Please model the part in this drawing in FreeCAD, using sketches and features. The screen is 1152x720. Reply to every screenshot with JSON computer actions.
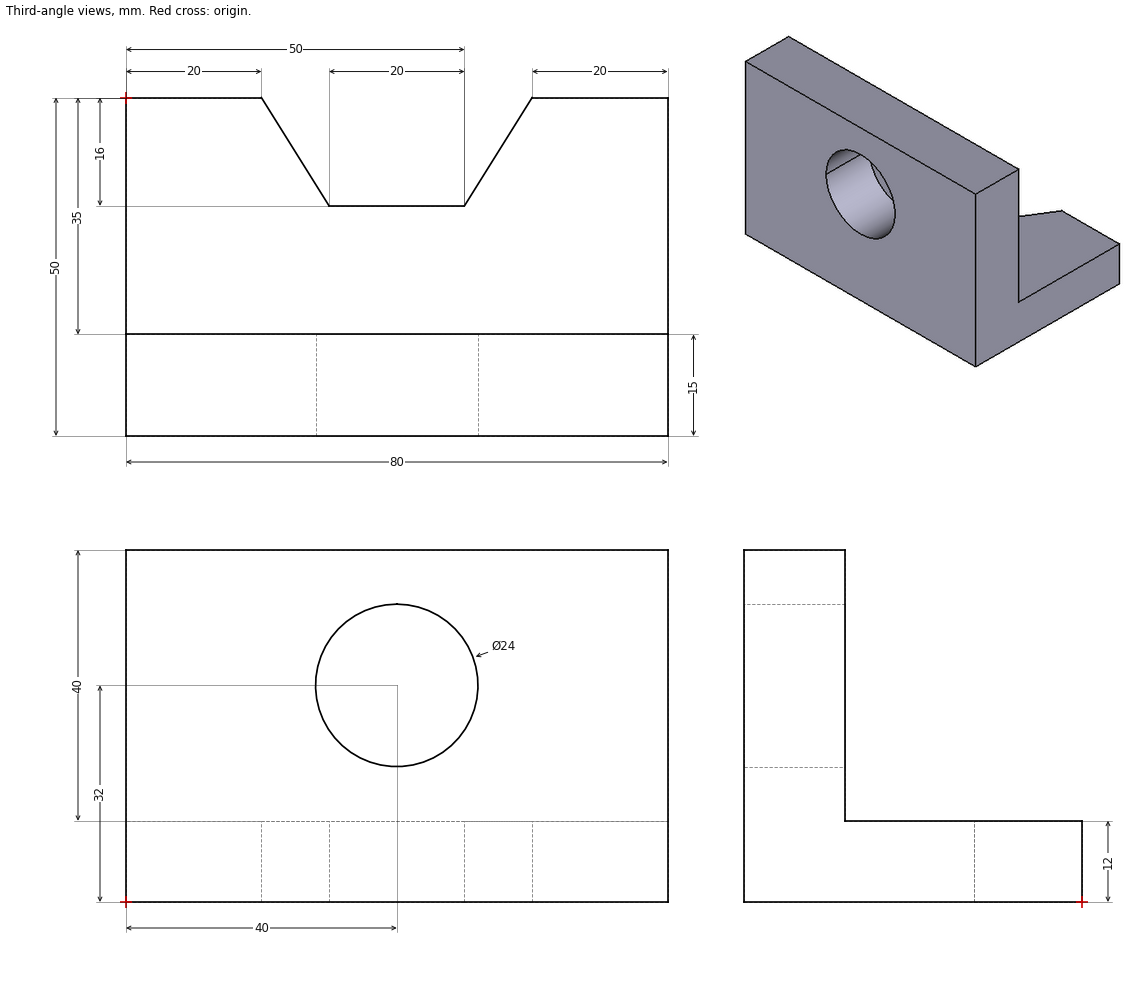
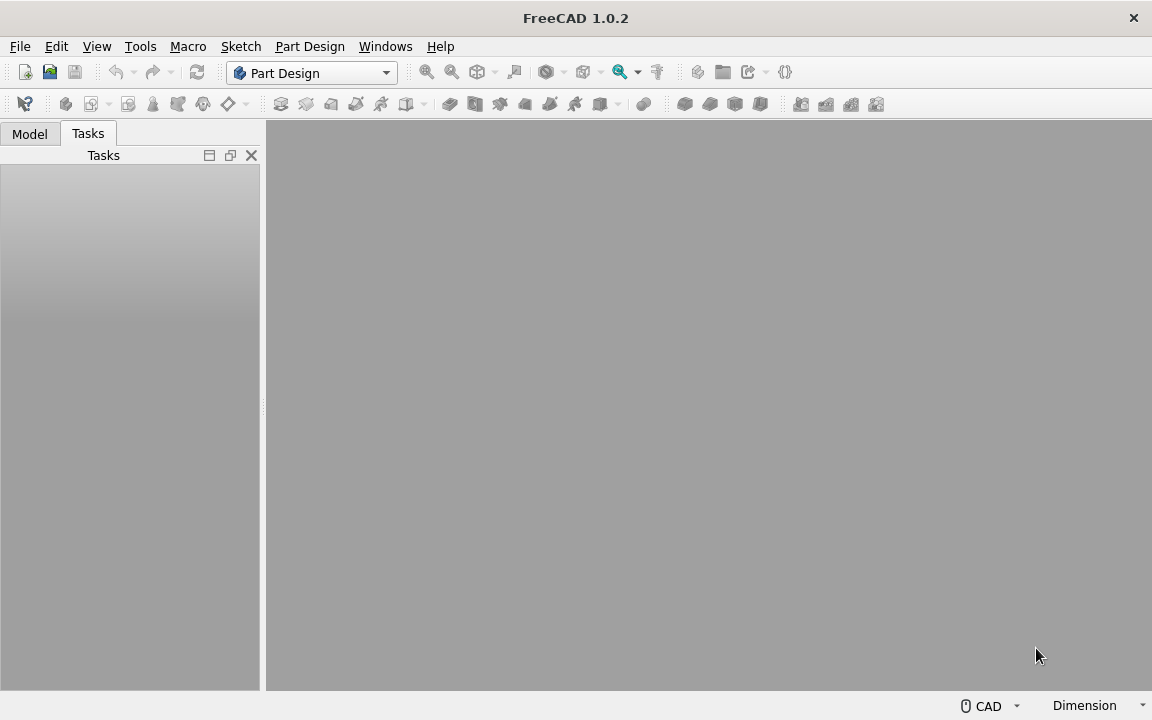
{"action": "key", "text": "ctrl+n"}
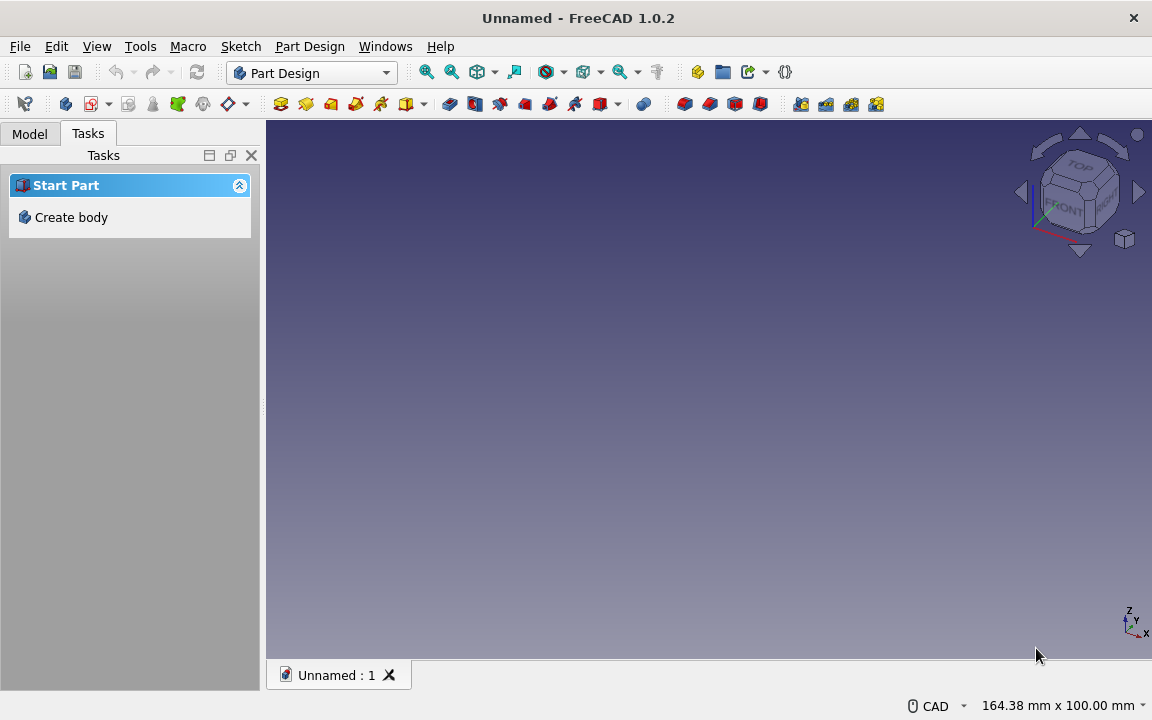
{"action": "left_click", "coordinate": [90, 104]}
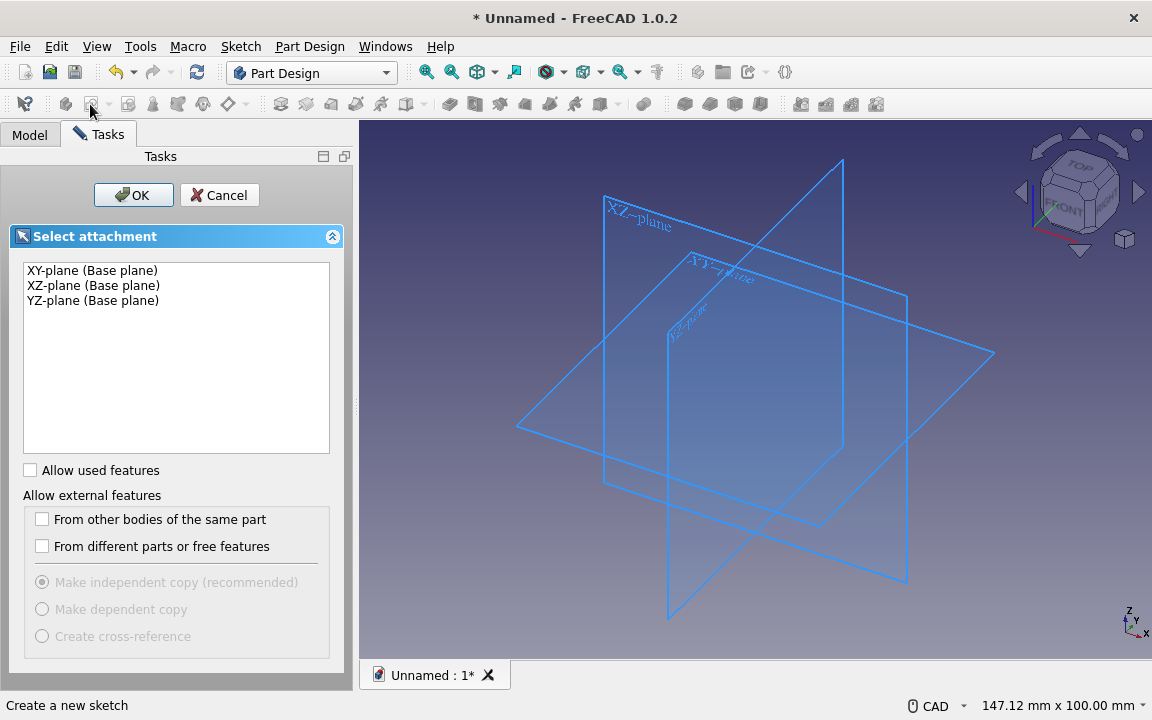
{"action": "left_click", "coordinate": [84, 270]}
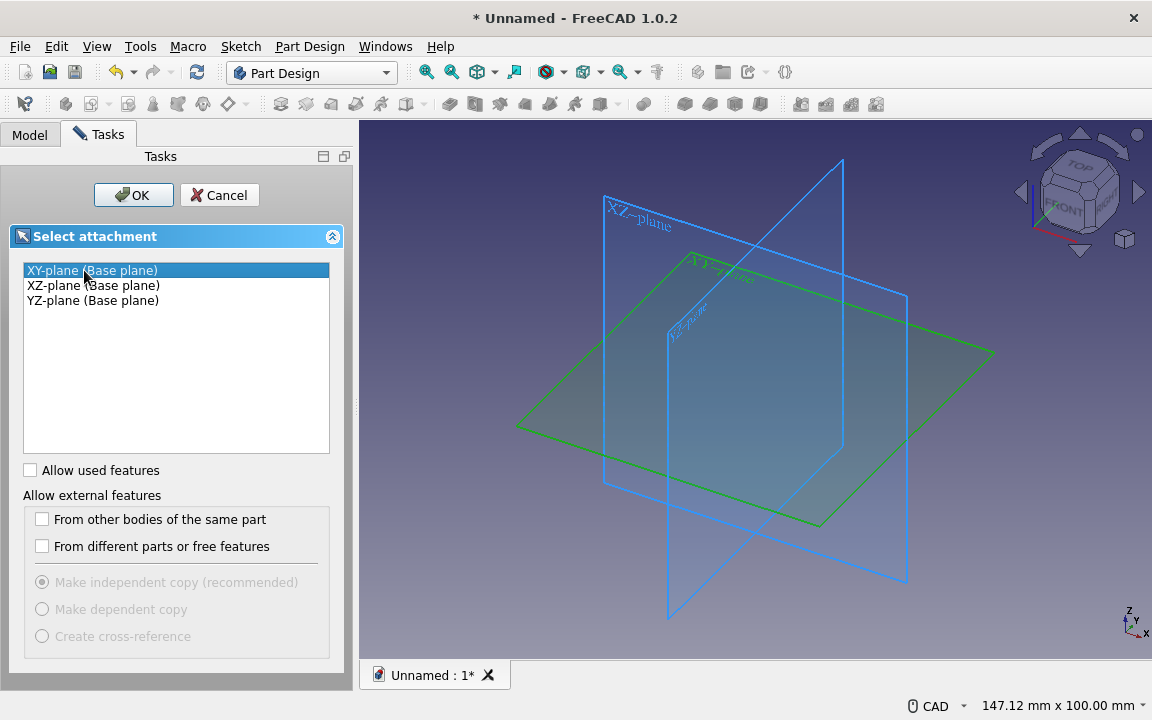
{"action": "left_click", "coordinate": [134, 195]}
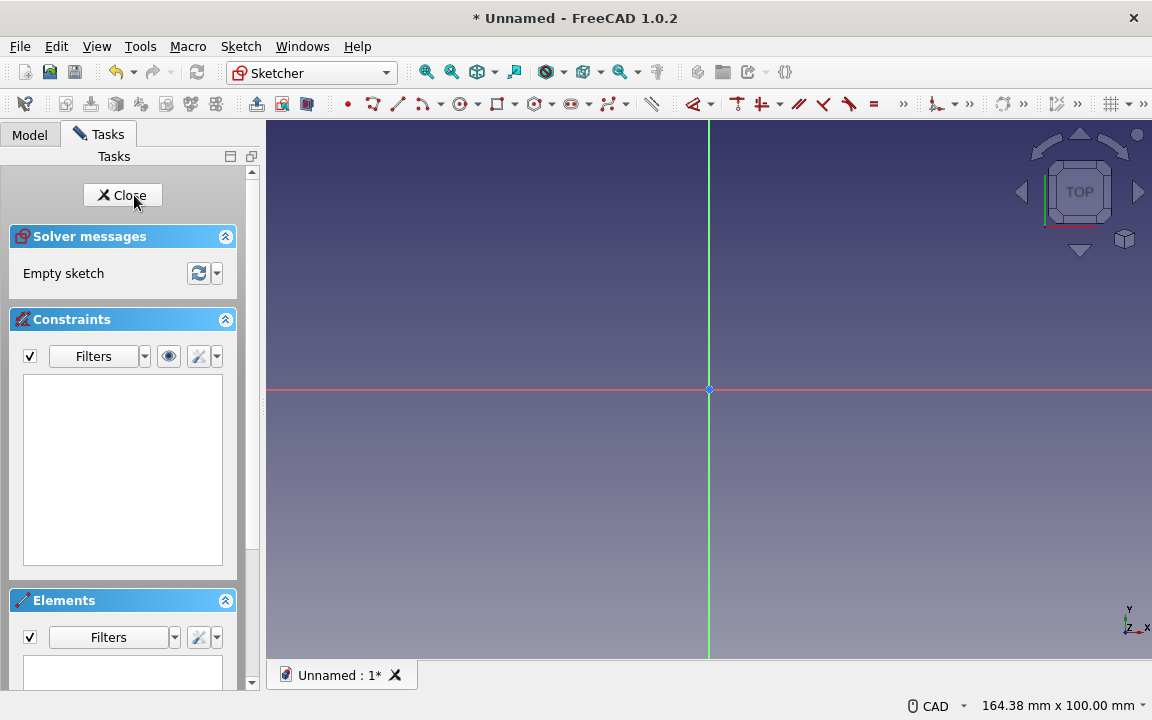
{"action": "scroll", "coordinate": [294, 148], "scroll_direction": "down", "scroll_amount": 2}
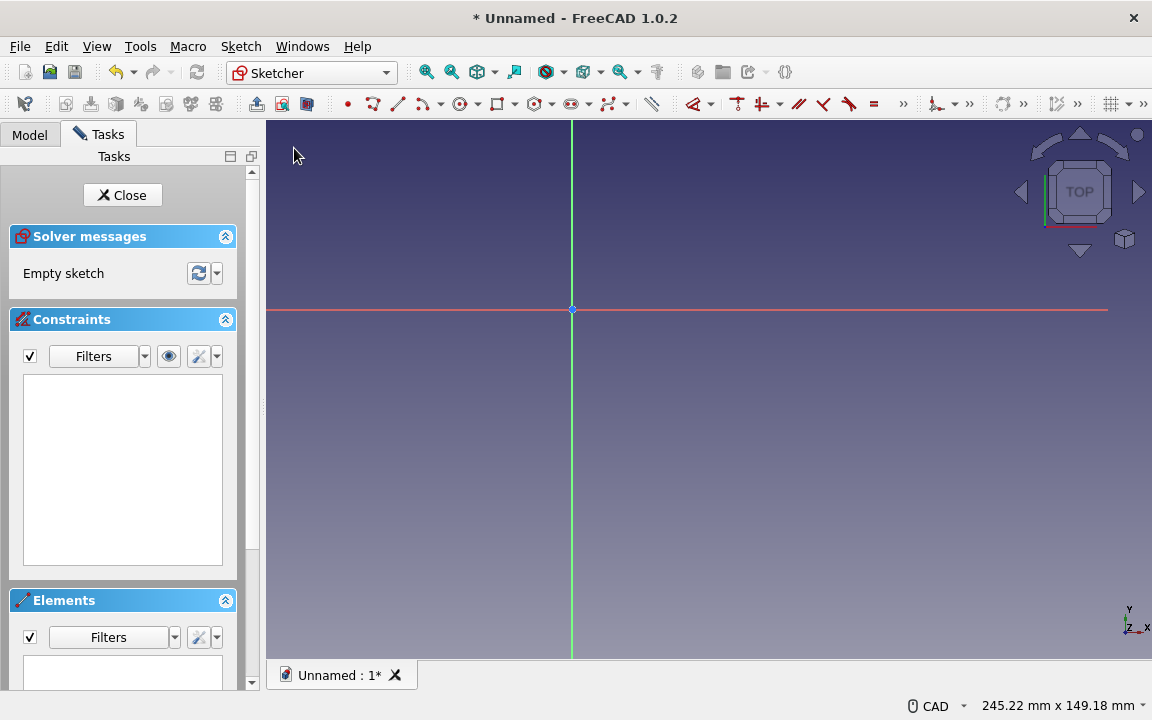
{"action": "scroll", "coordinate": [809, 413], "scroll_direction": "up", "scroll_amount": 3}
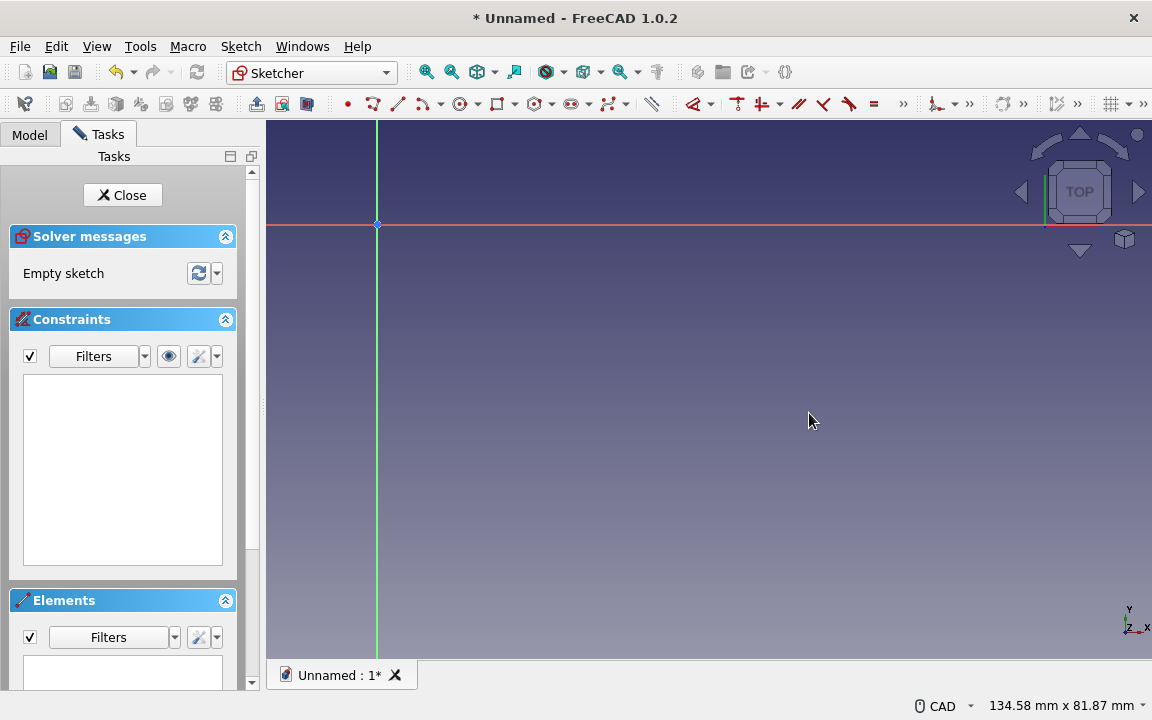
{"action": "left_click", "coordinate": [373, 104]}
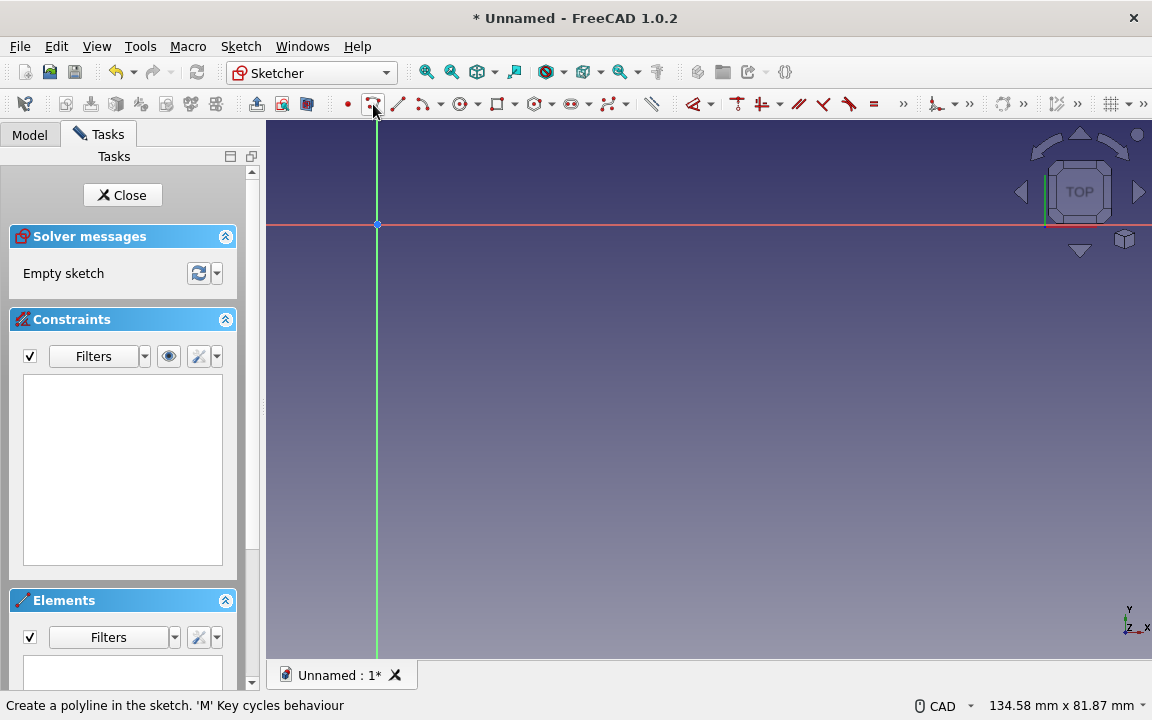
{"action": "left_click", "coordinate": [377, 225]}
{"action": "left_click", "coordinate": [386, 554]}
{"action": "left_click", "coordinate": [904, 554]}
{"action": "left_click", "coordinate": [904, 225]}
{"action": "left_click", "coordinate": [772, 234]}
{"action": "left_click", "coordinate": [706, 330]}
{"action": "left_click", "coordinate": [575, 330]}
{"action": "left_click", "coordinate": [509, 234]}
{"action": "left_click", "coordinate": [377, 225]}
{"action": "key", "text": "Escape"}
{"action": "key", "text": "Escape"}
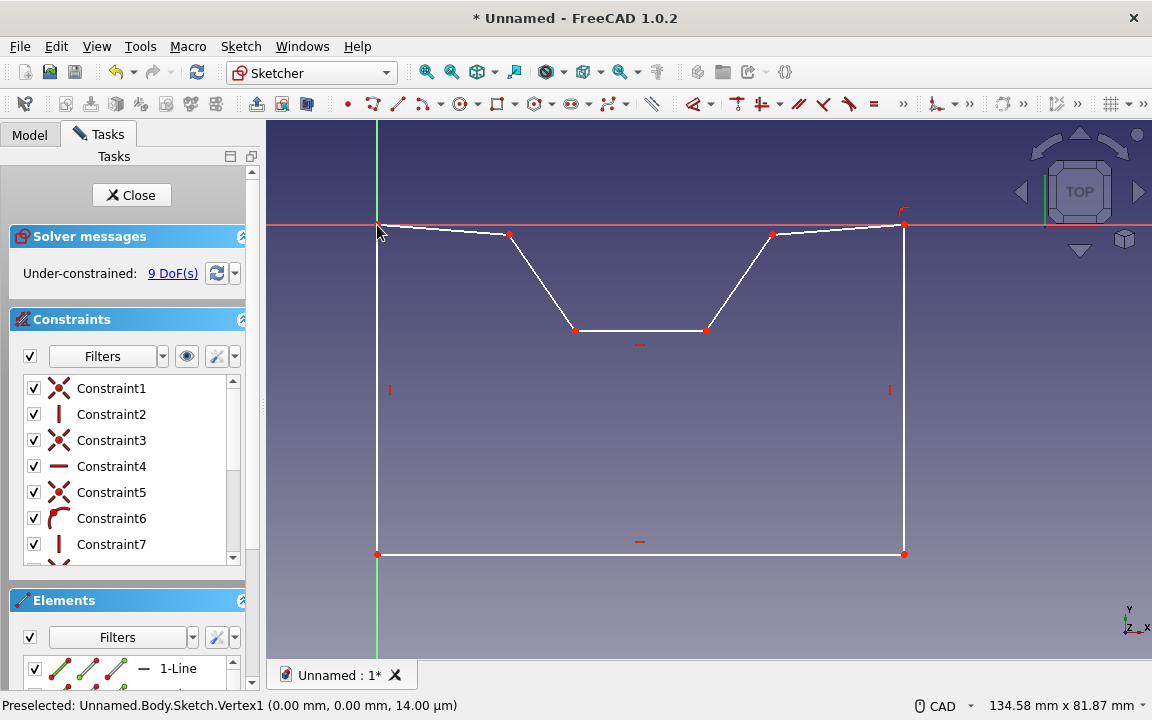
{"action": "left_click", "coordinate": [864, 228]}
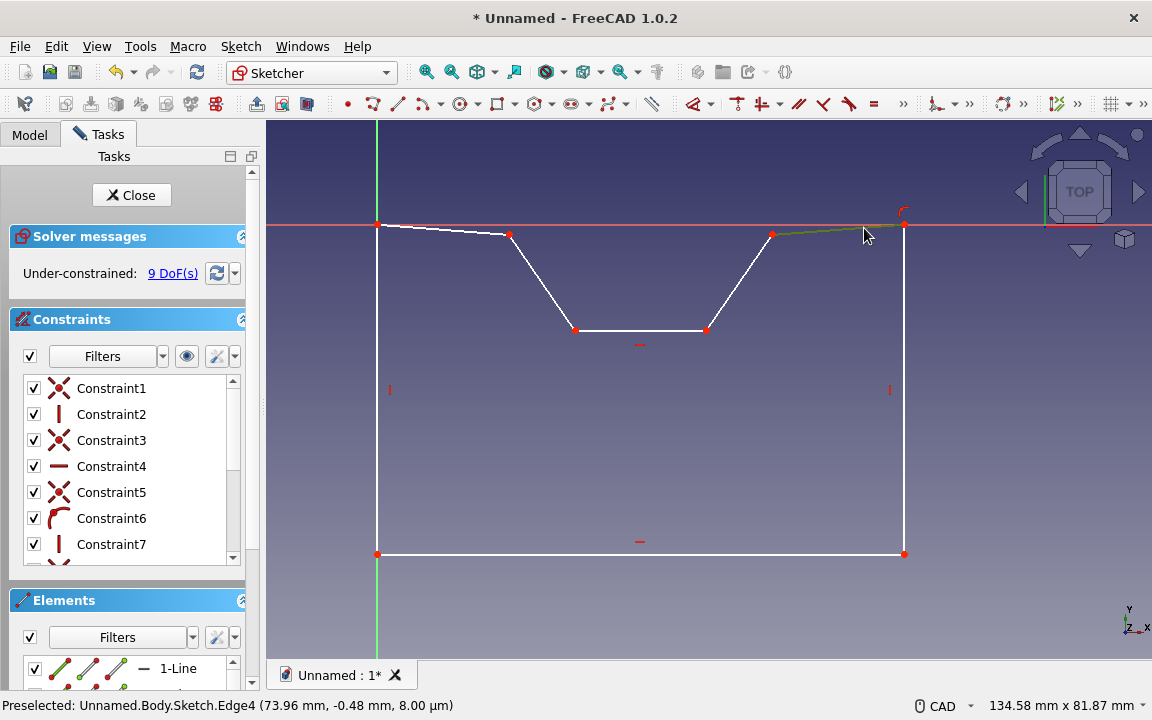
{"action": "left_click", "coordinate": [780, 104]}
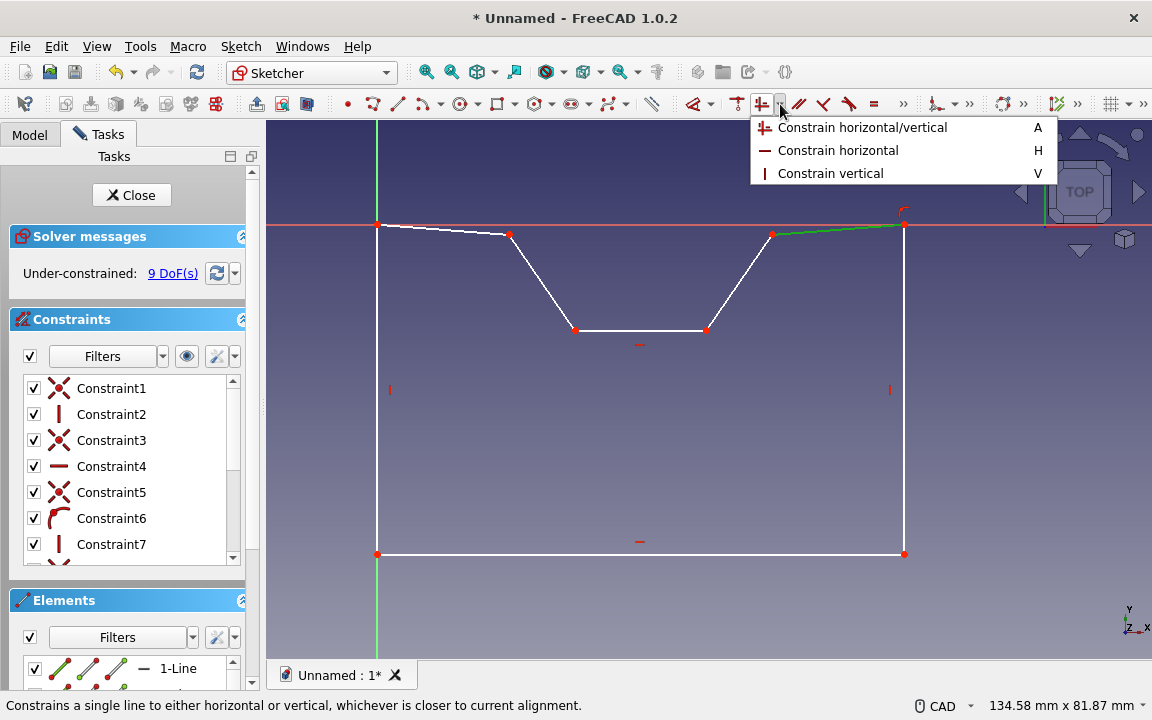
{"action": "left_click", "coordinate": [904, 150]}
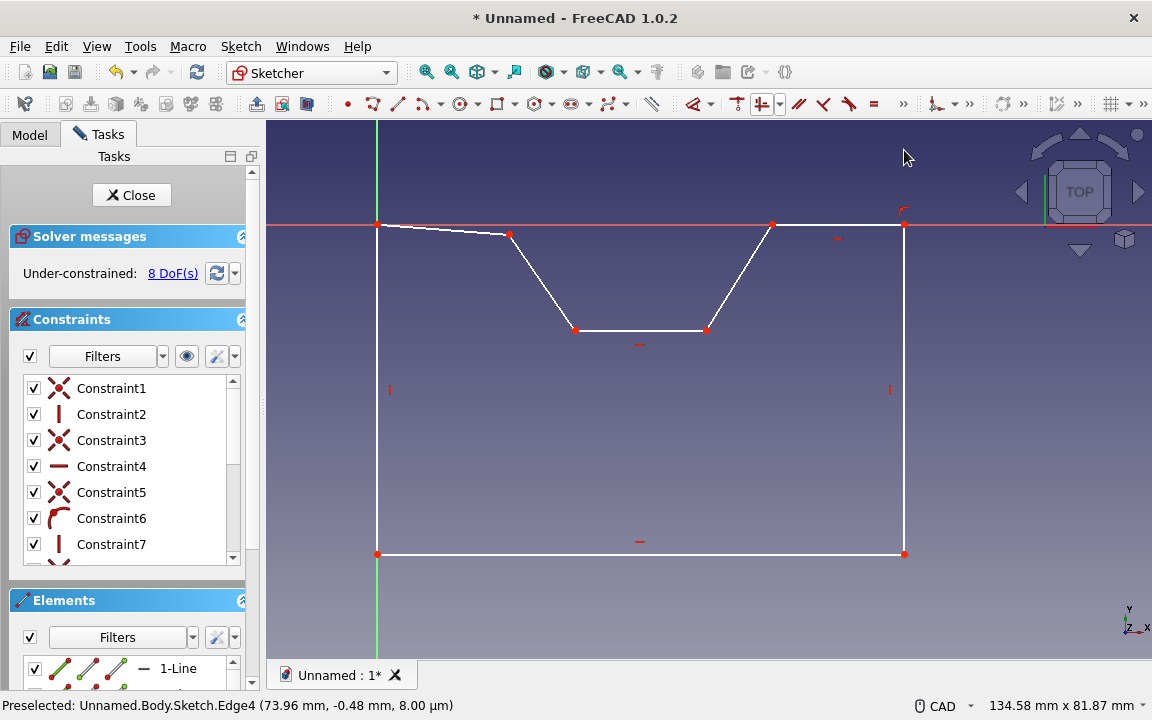
{"action": "left_click", "coordinate": [417, 228]}